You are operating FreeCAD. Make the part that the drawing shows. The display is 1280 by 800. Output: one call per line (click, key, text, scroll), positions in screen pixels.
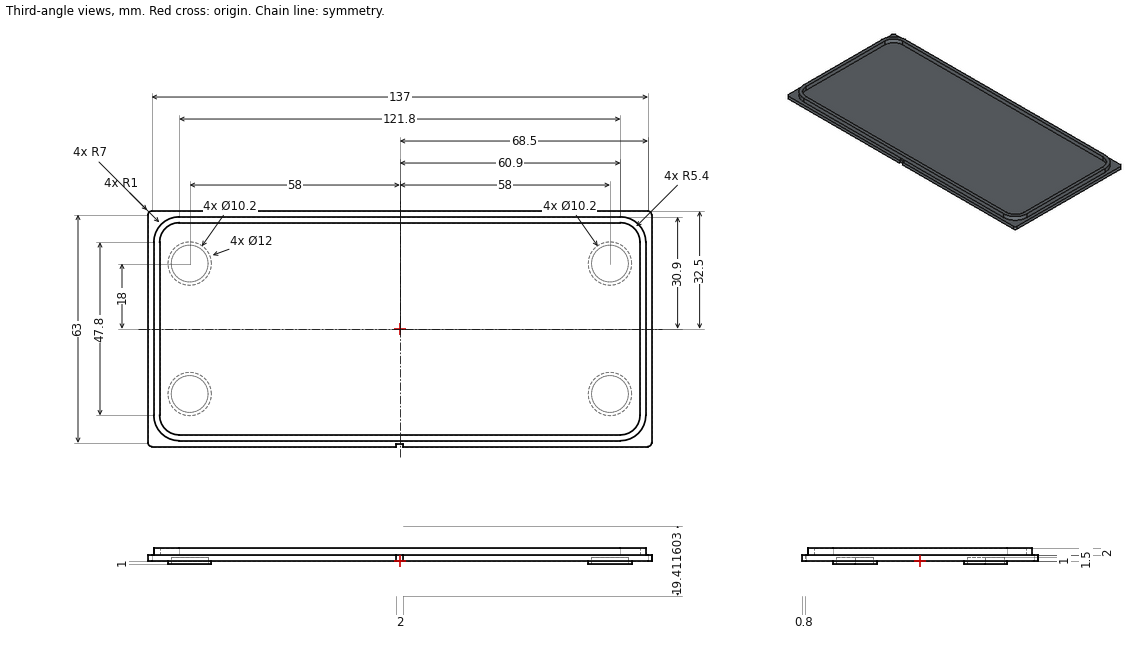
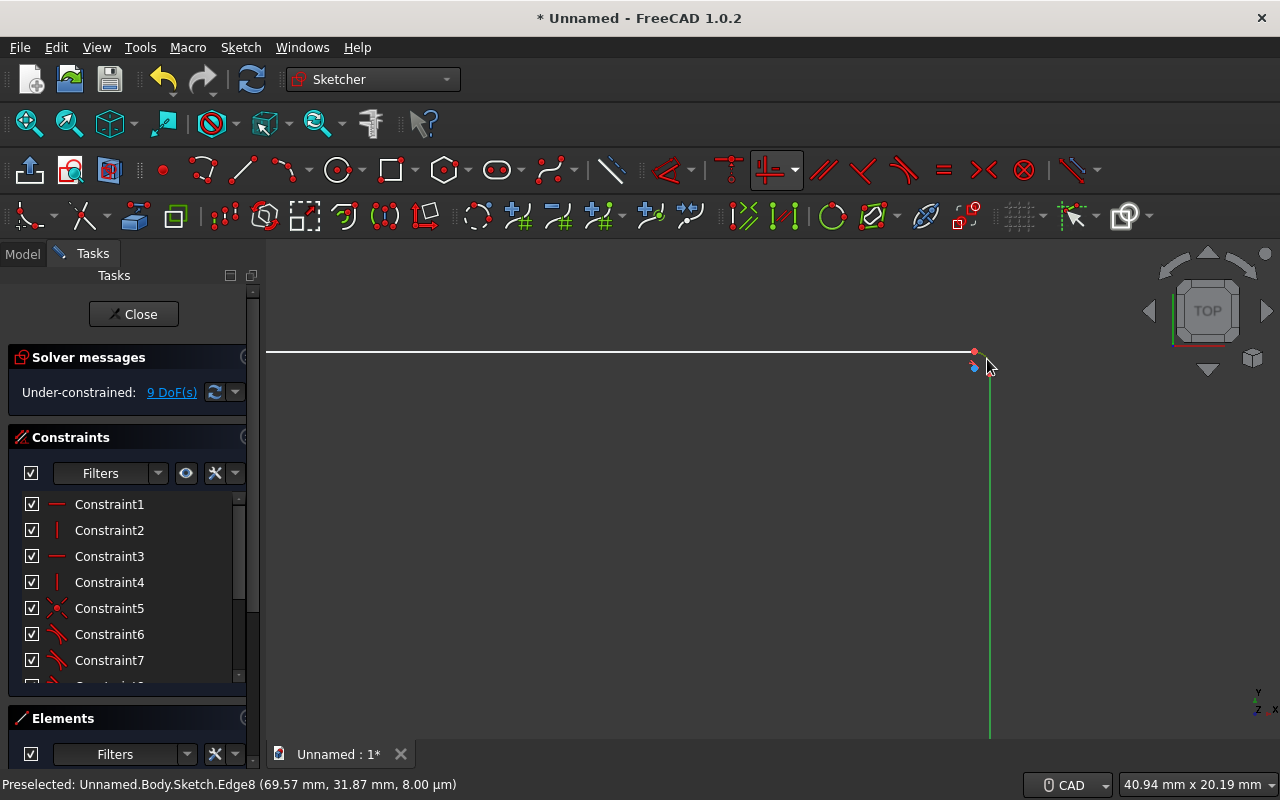
click(904, 170)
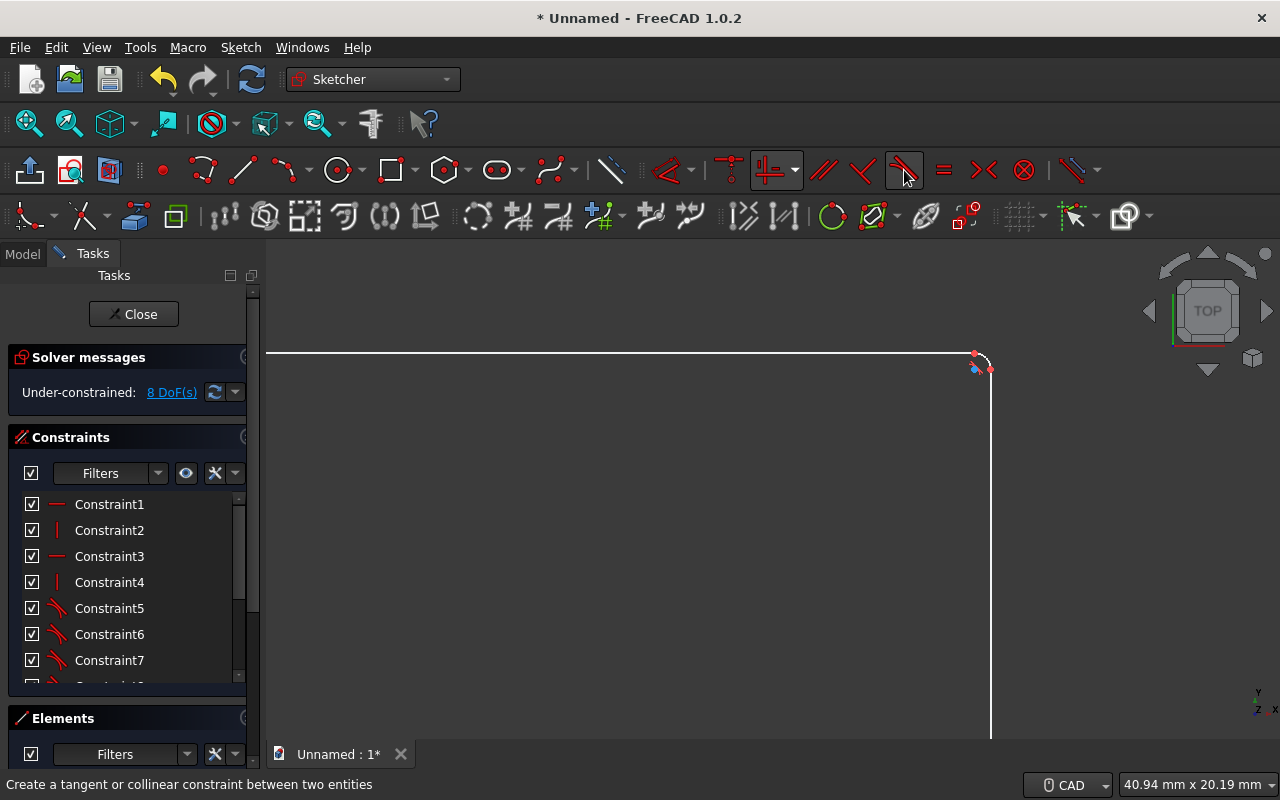
scroll(989, 358, down, 9)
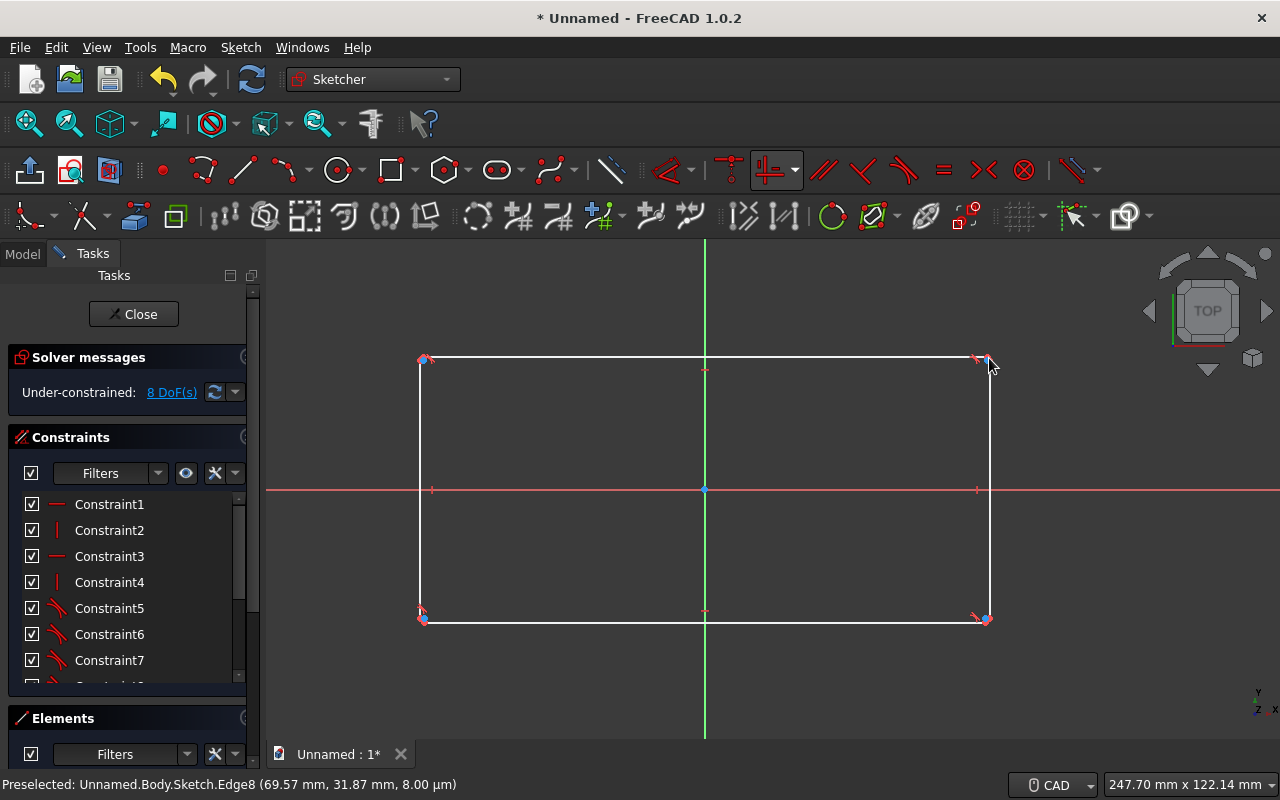
scroll(421, 358, up, 10)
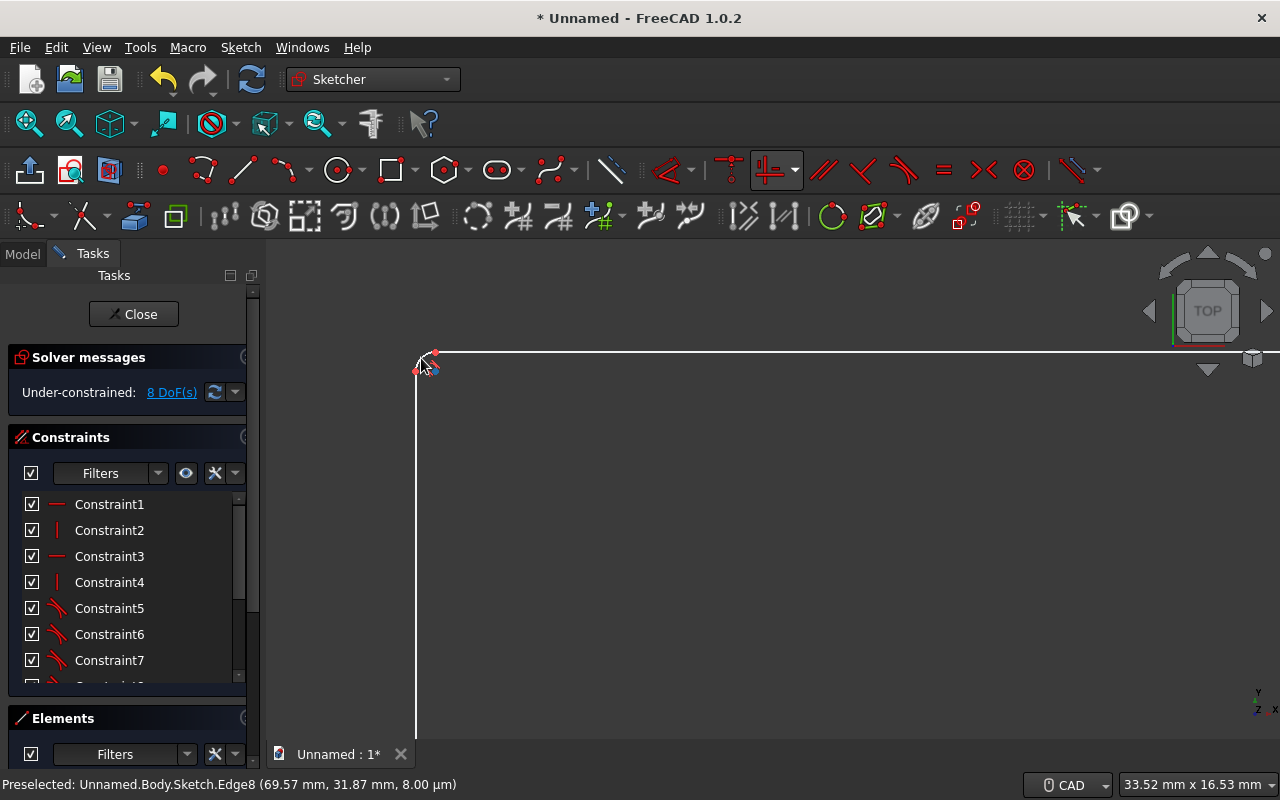
click(422, 358)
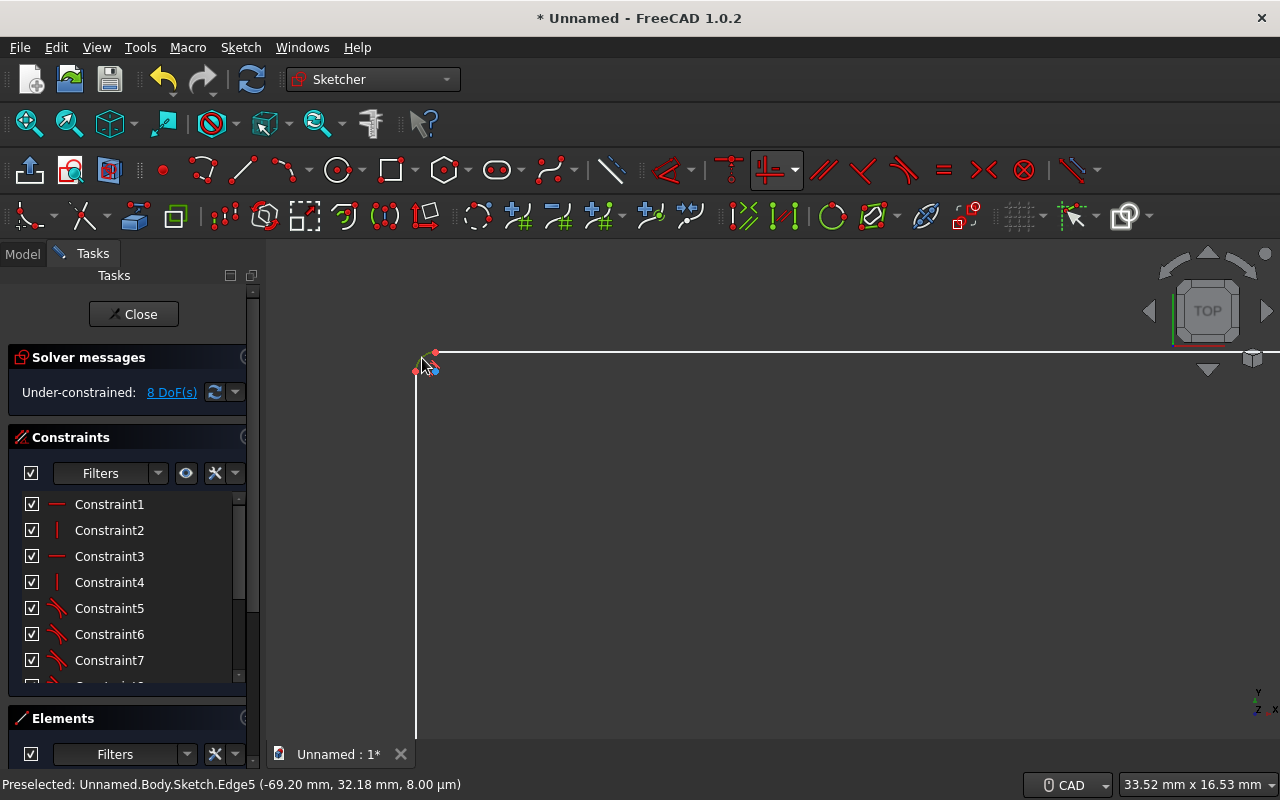
scroll(421, 358, down, 10)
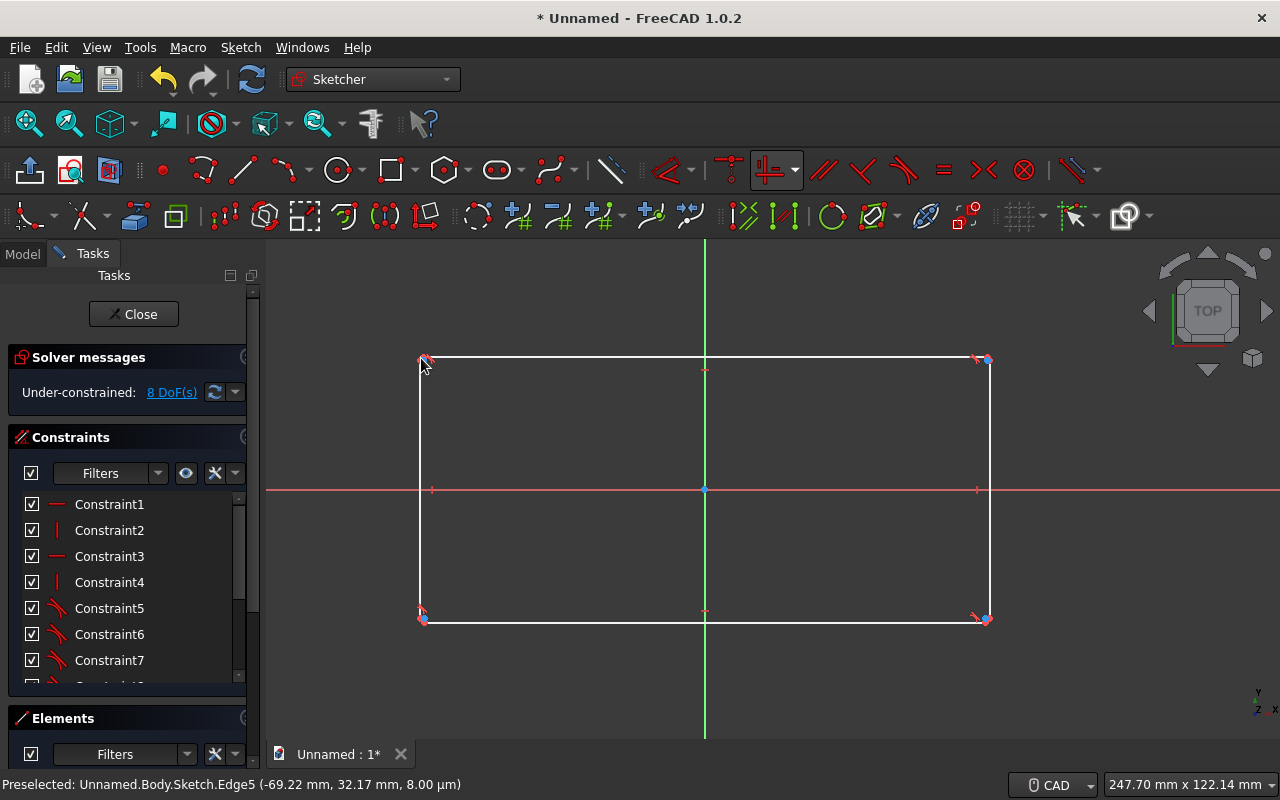
scroll(421, 620, up, 10)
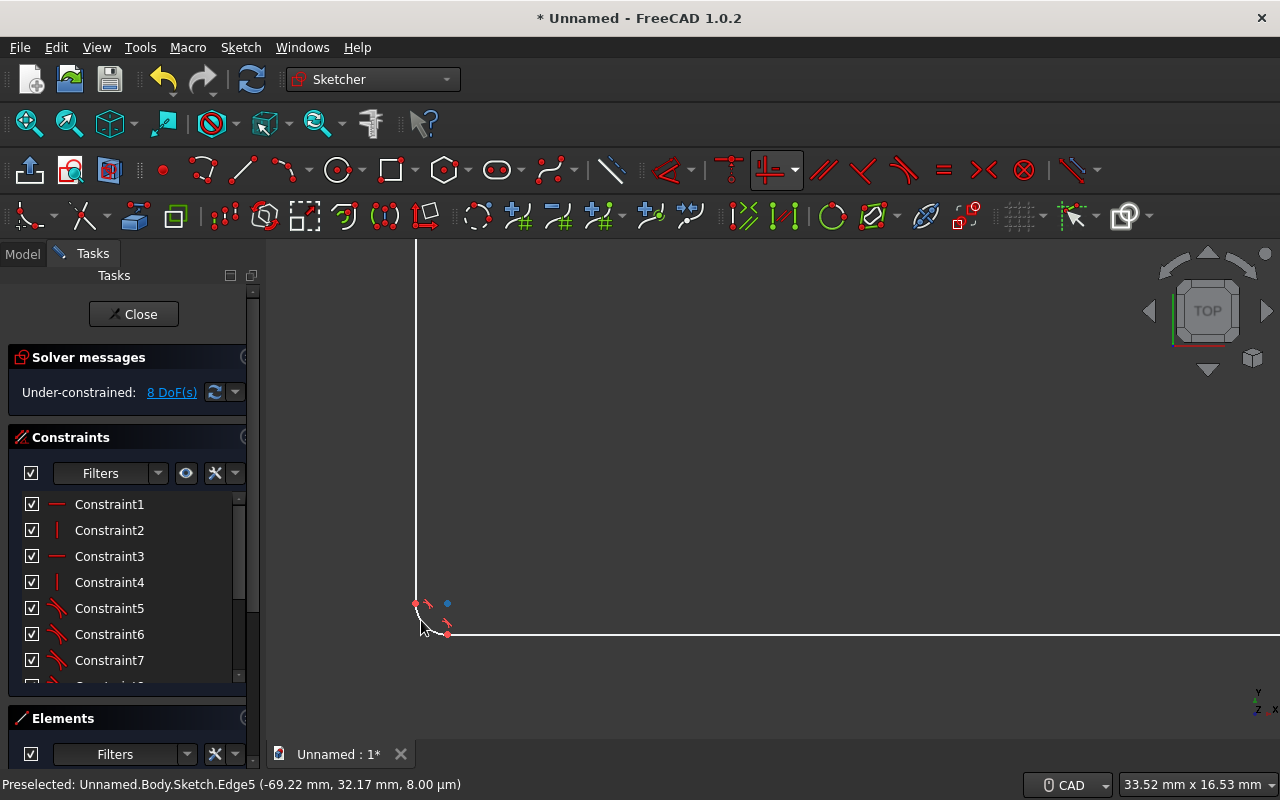
click(419, 618)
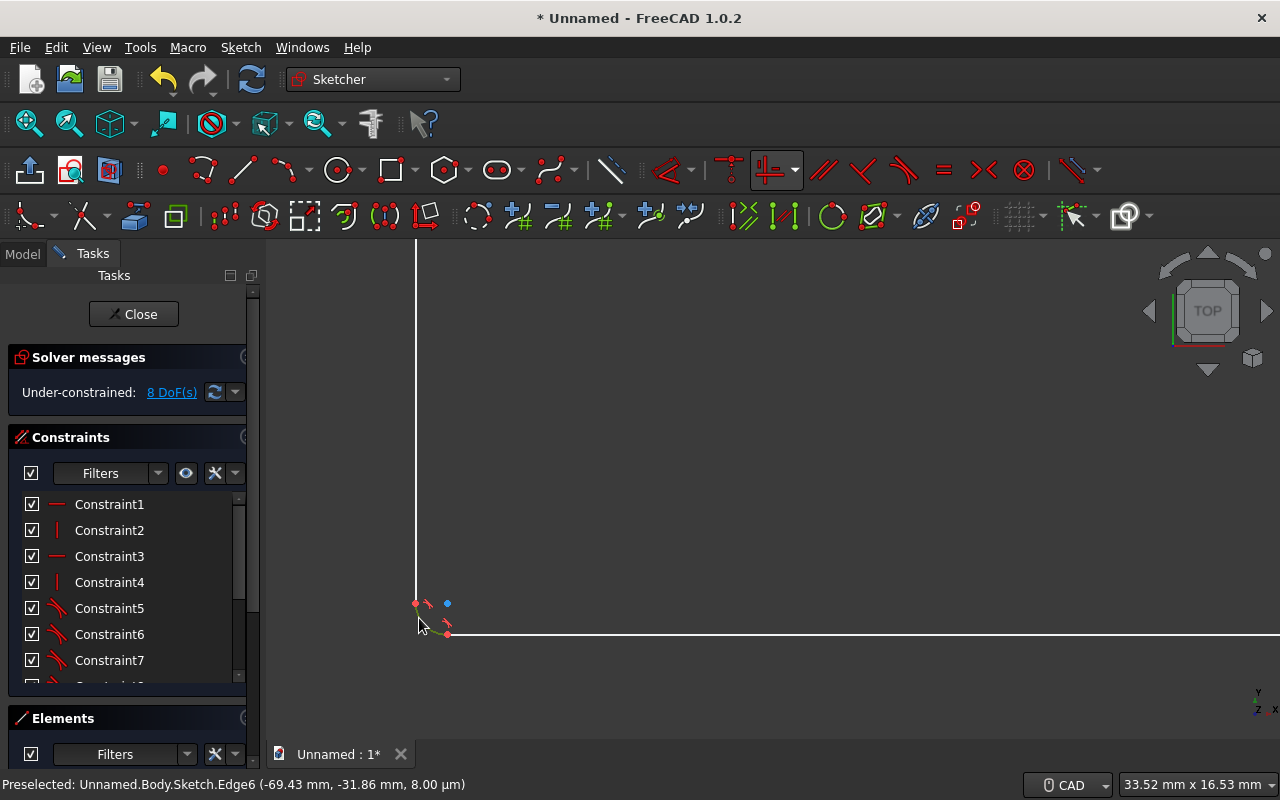
scroll(421, 620, down, 10)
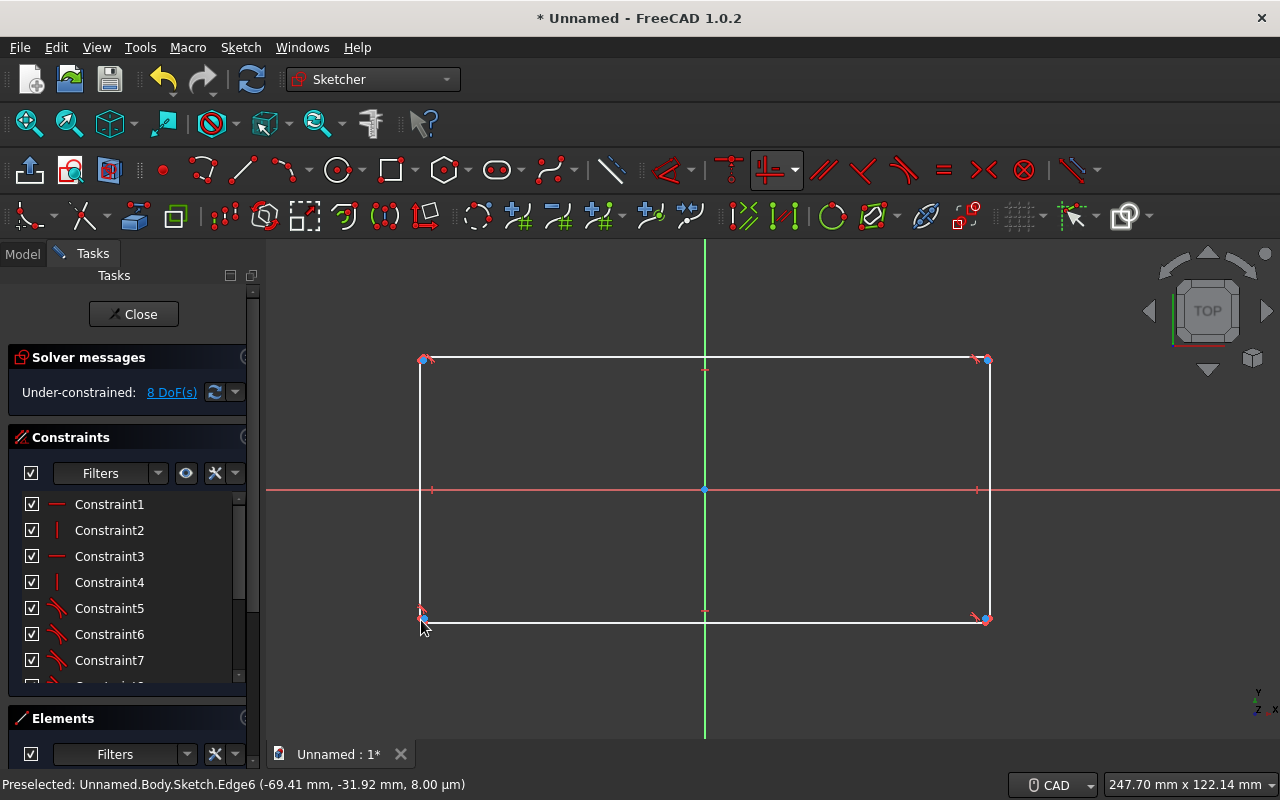
scroll(987, 622, up, 10)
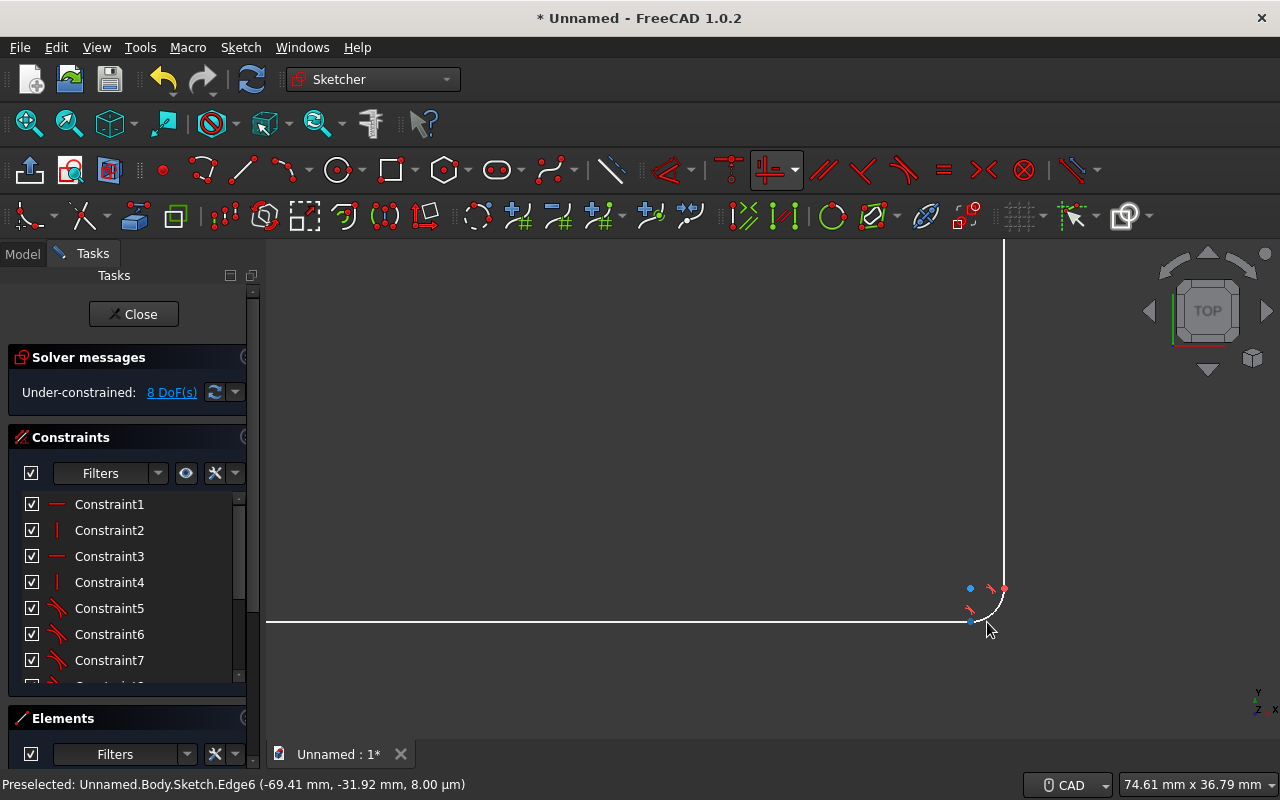
click(986, 618)